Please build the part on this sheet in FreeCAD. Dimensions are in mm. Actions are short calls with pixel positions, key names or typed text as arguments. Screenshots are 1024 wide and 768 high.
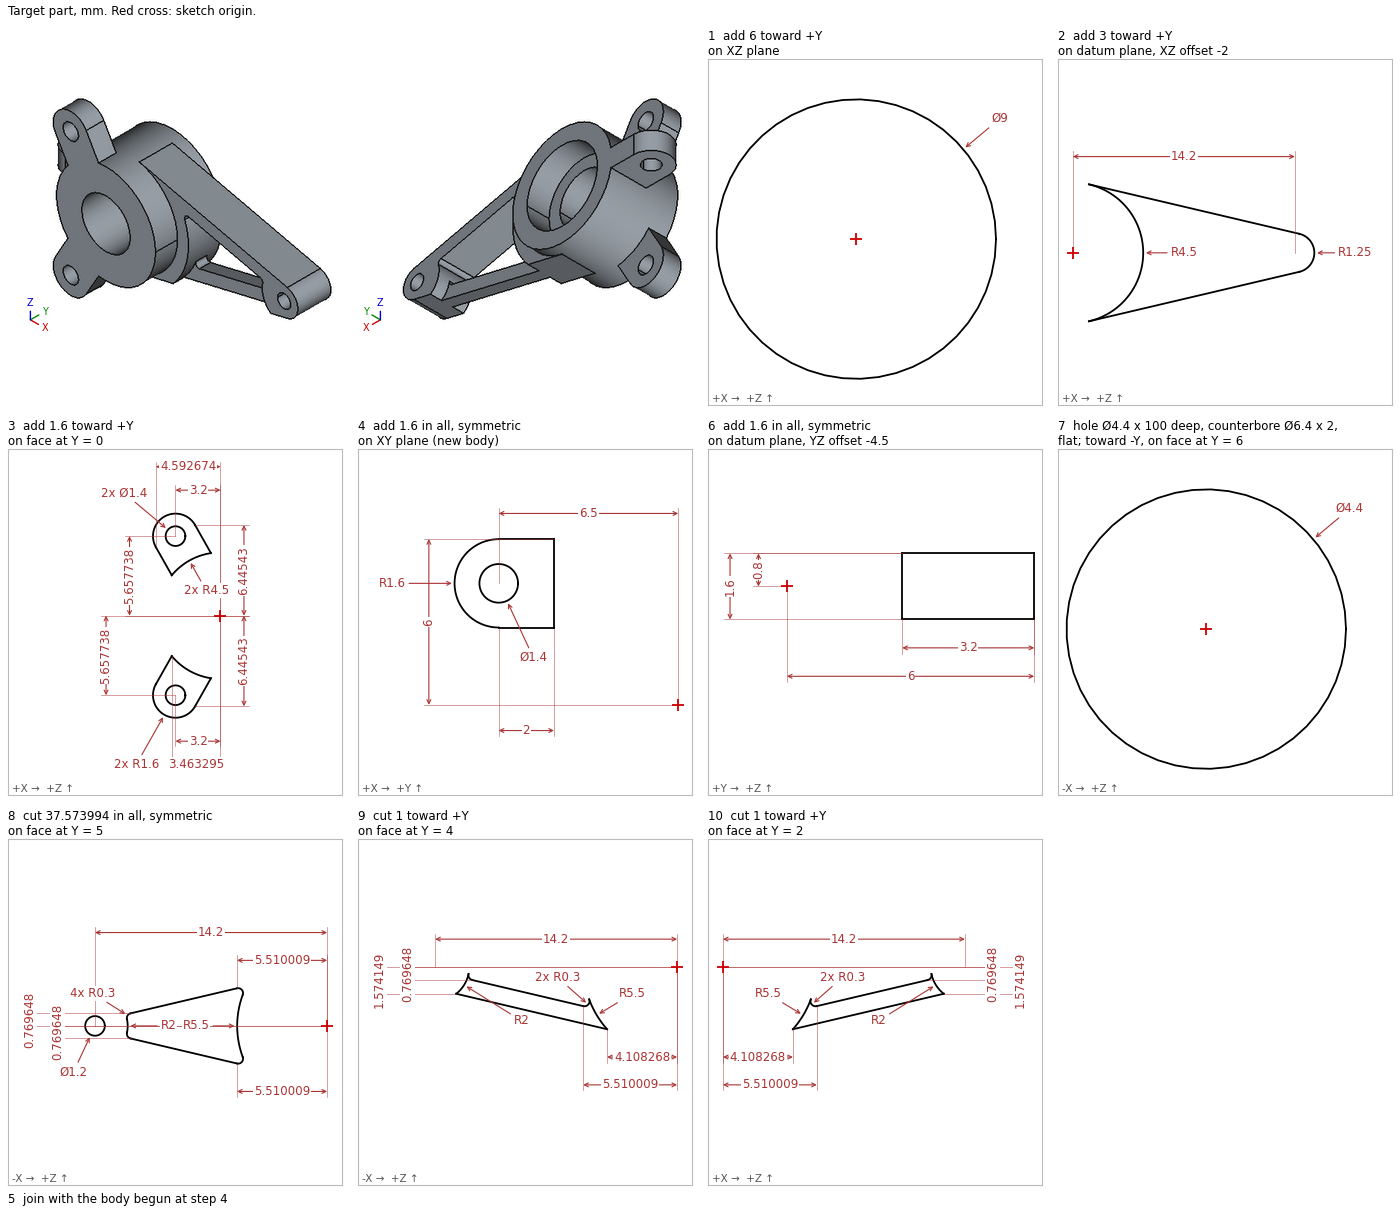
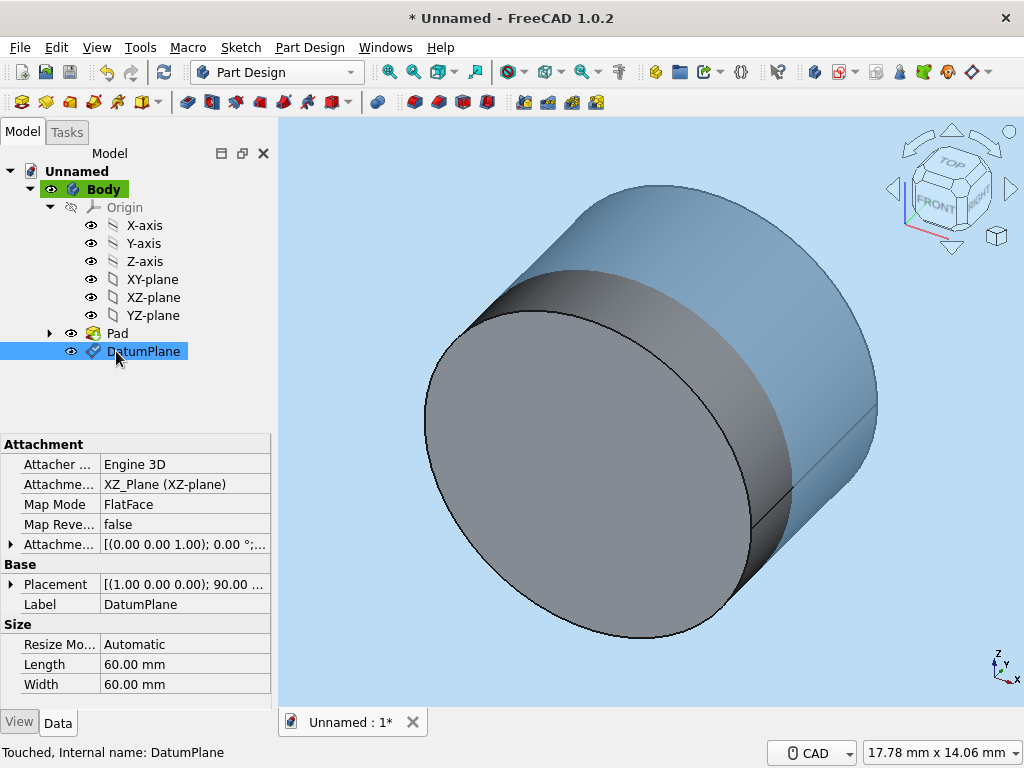
click(840, 72)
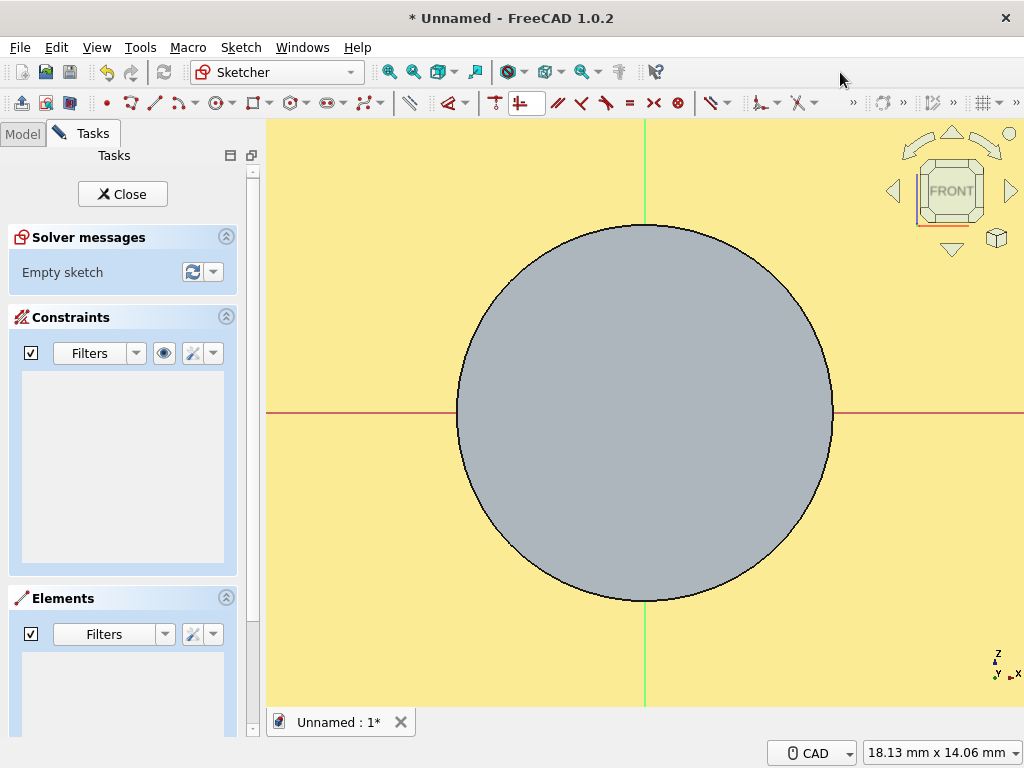
click(70, 104)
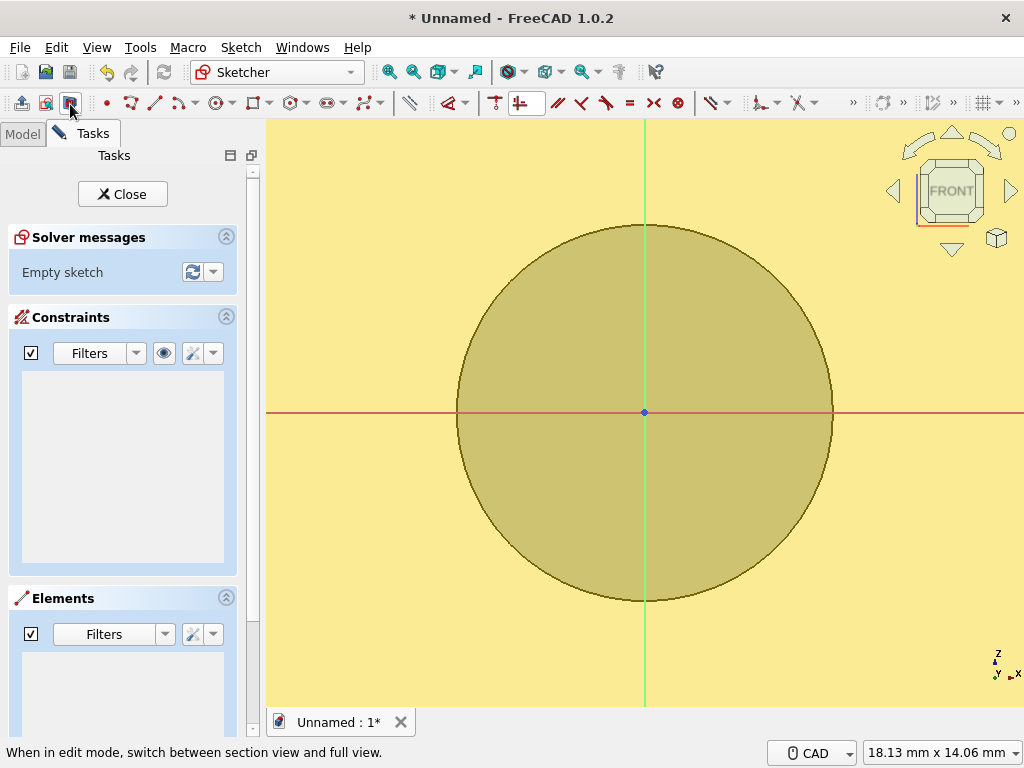
scroll(294, 413, down, 4)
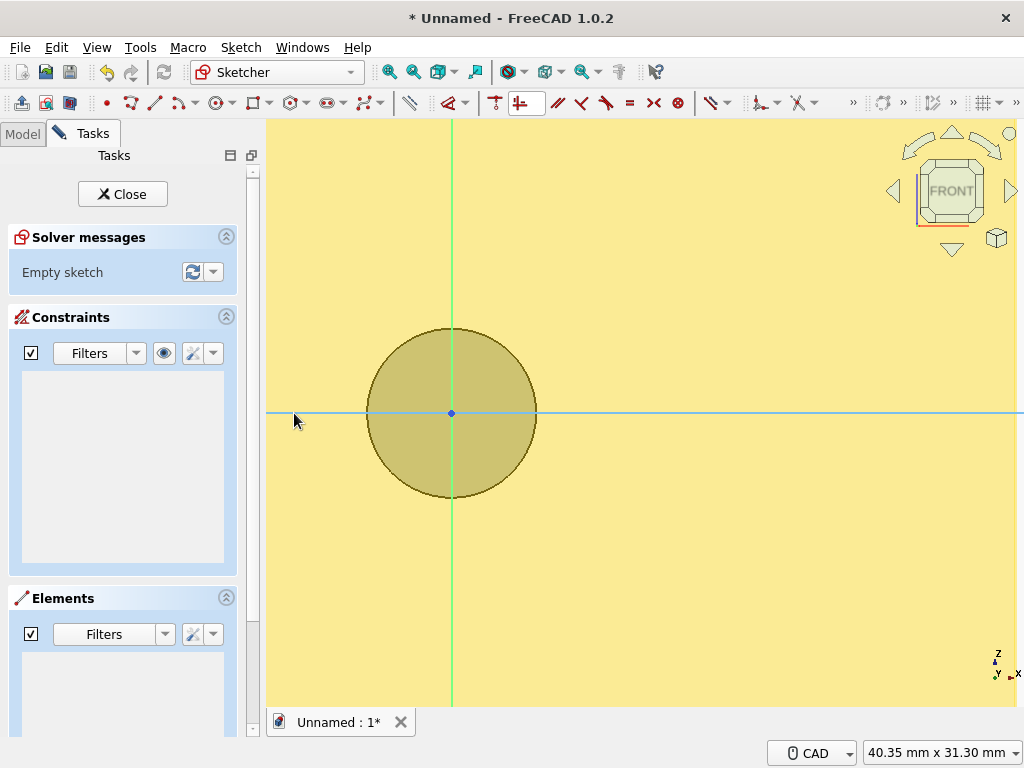
scroll(638, 414, up, 2)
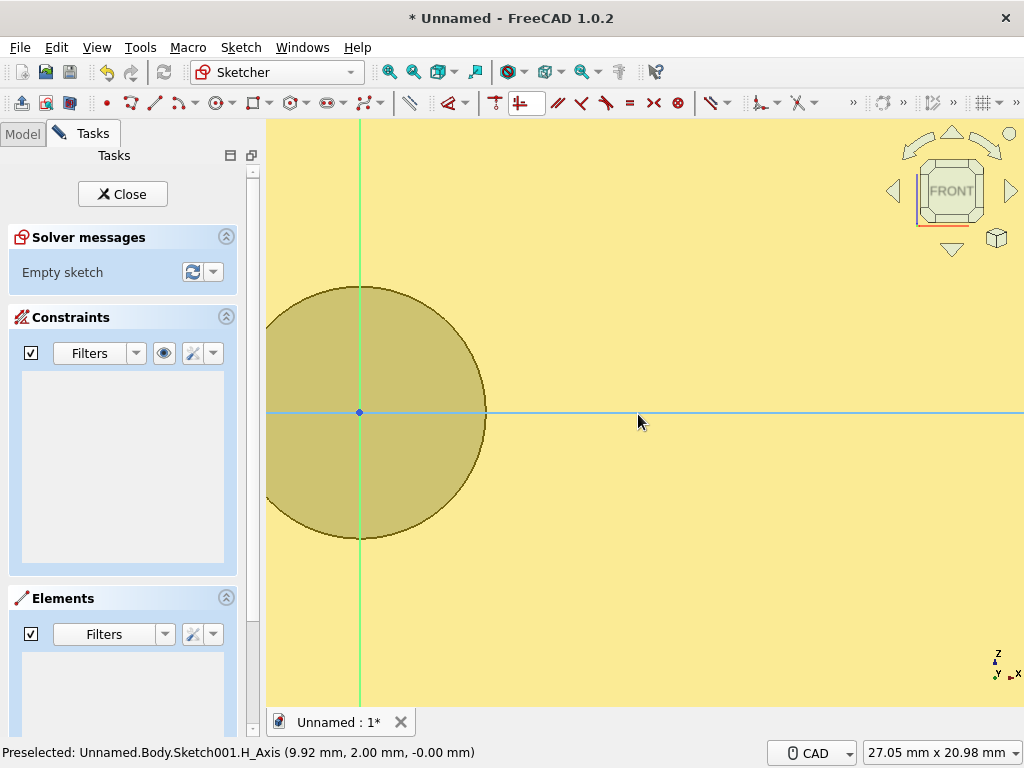
key(g)
key(l)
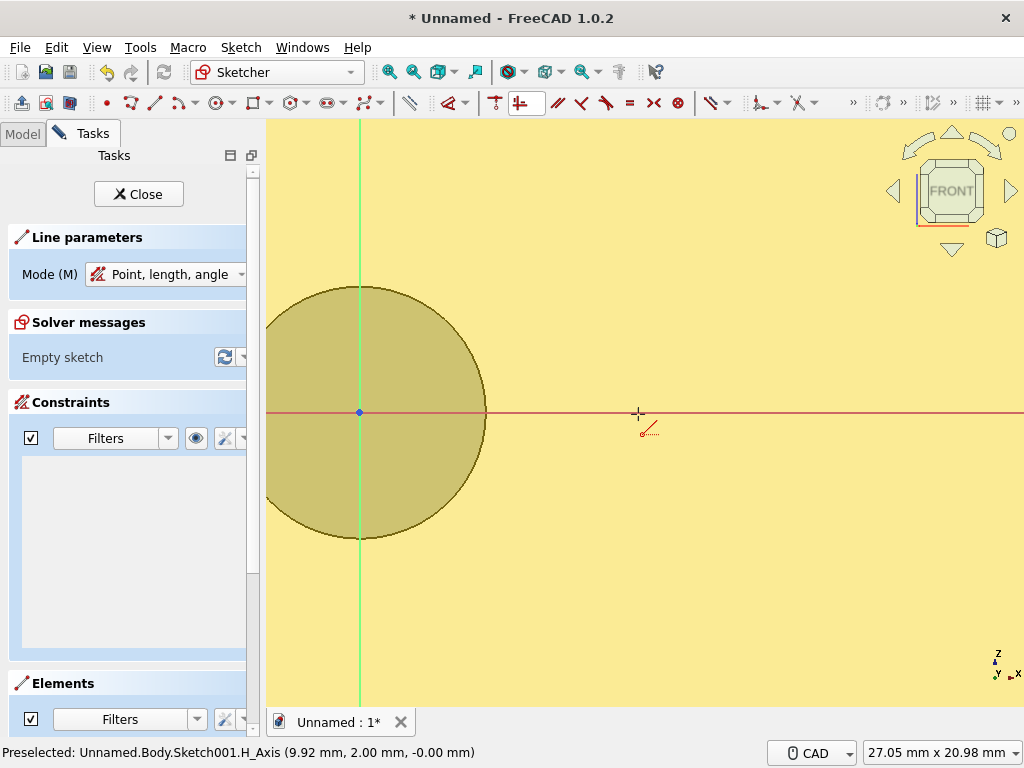
click(766, 447)
click(389, 535)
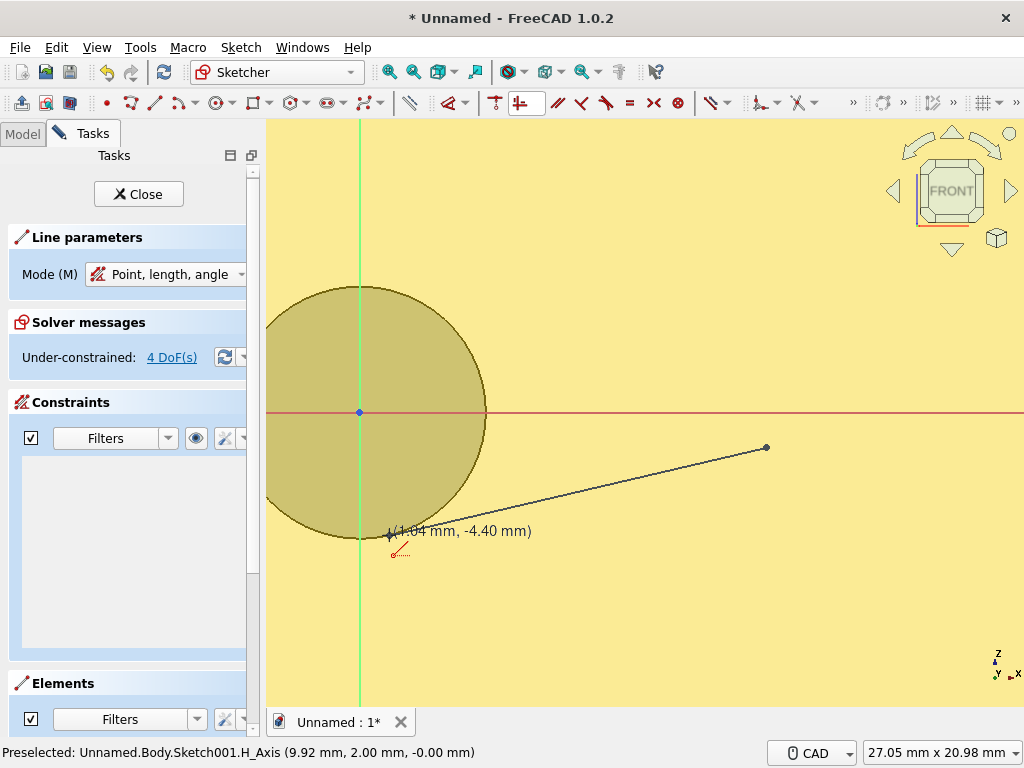
click(389, 290)
click(766, 379)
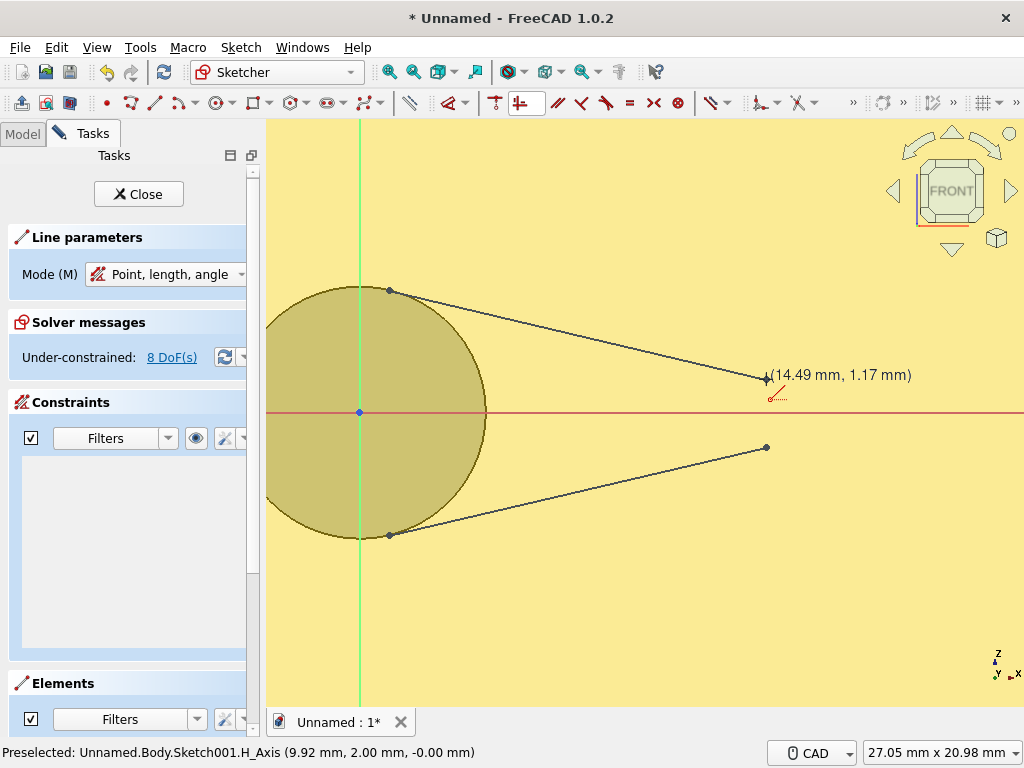
key(g)
key(3)
key(a)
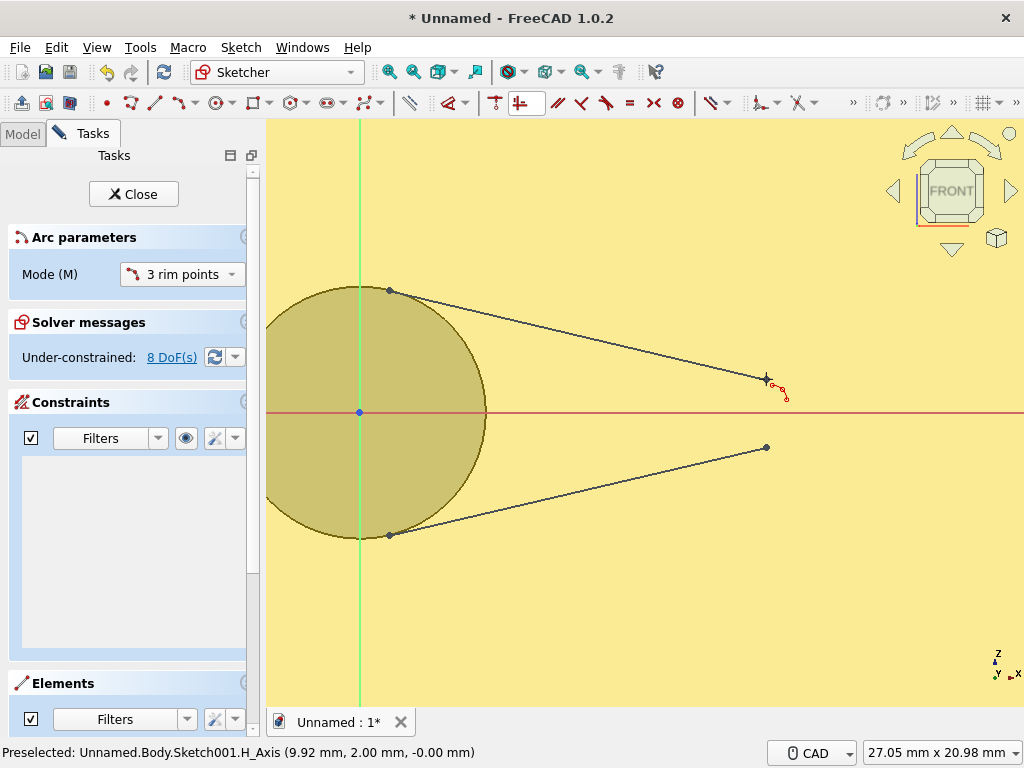
click(389, 536)
click(389, 291)
click(481, 446)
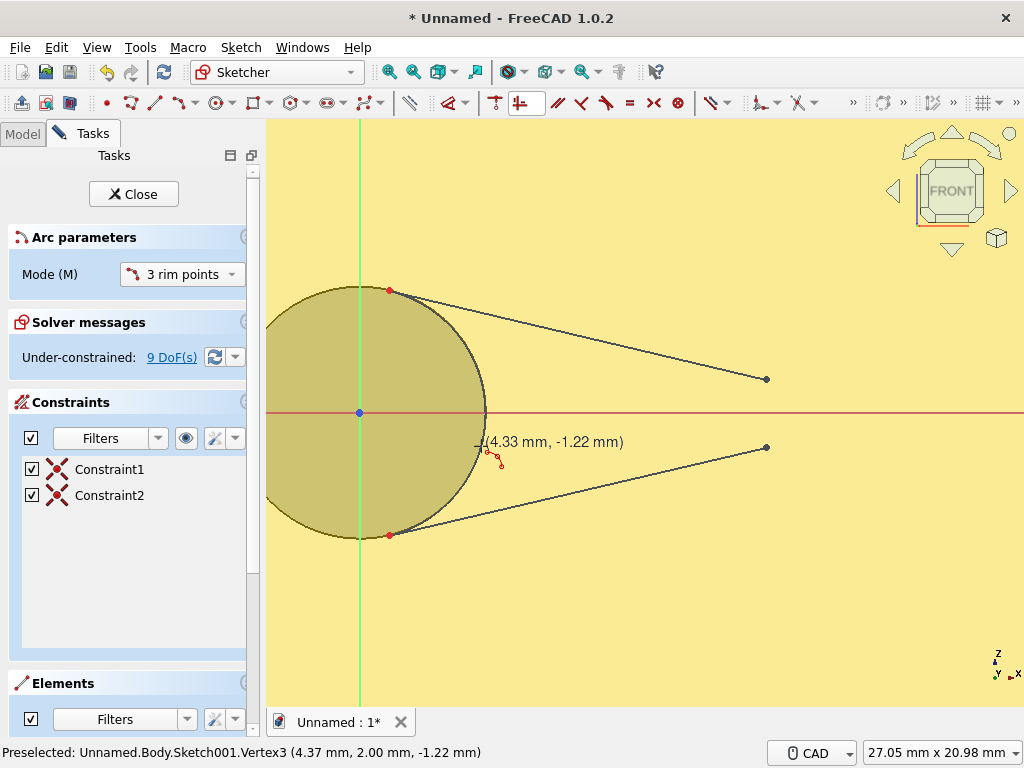
click(766, 380)
click(766, 448)
click(788, 431)
key(Escape)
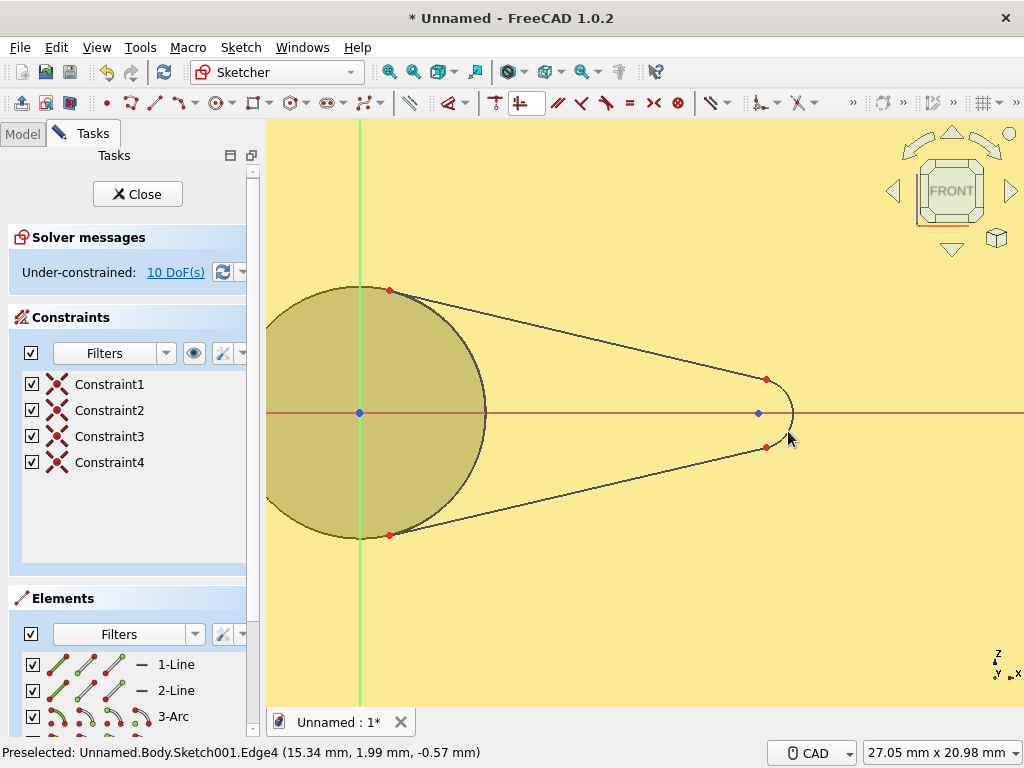
click(653, 474)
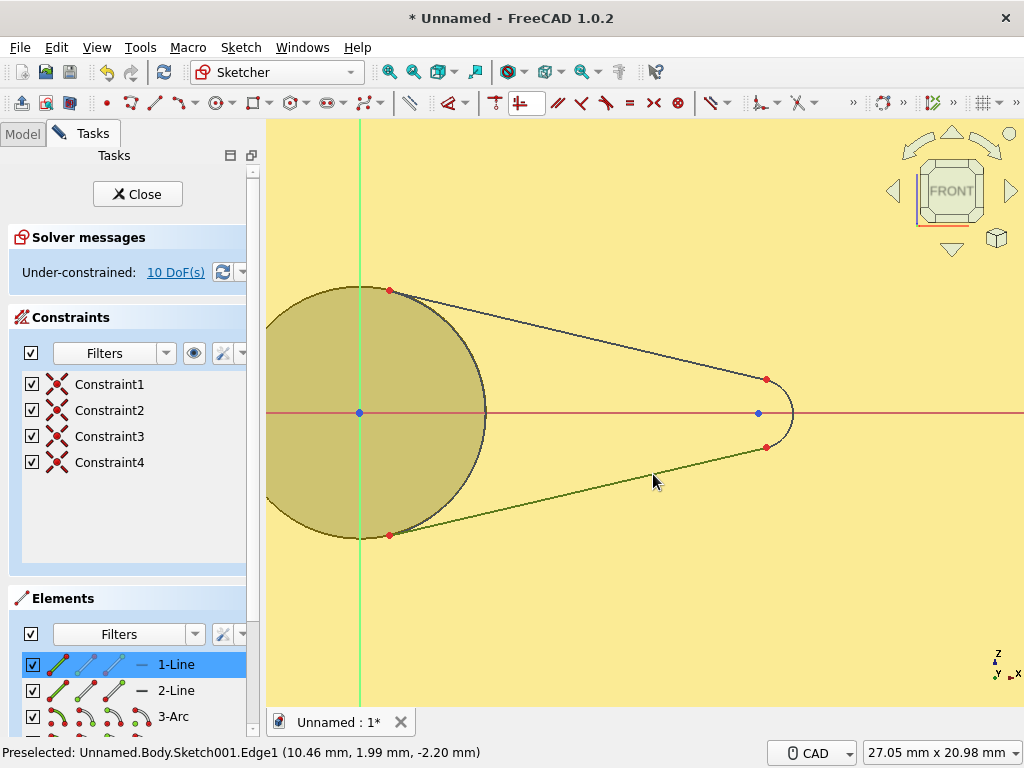
click(468, 478)